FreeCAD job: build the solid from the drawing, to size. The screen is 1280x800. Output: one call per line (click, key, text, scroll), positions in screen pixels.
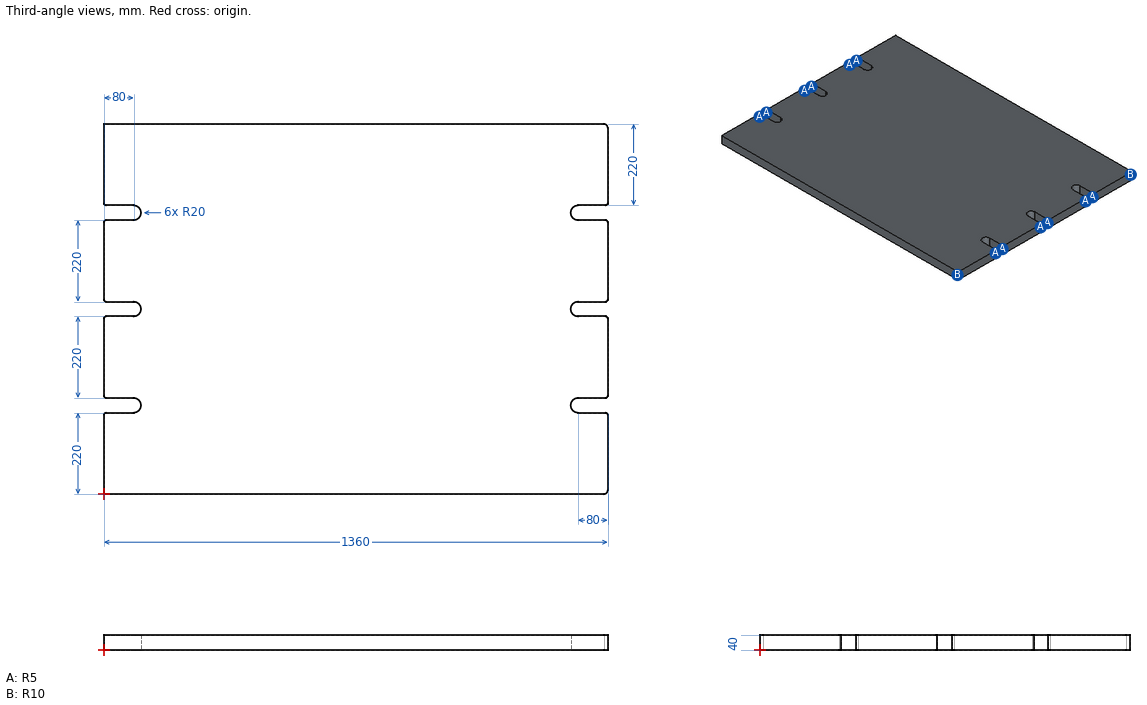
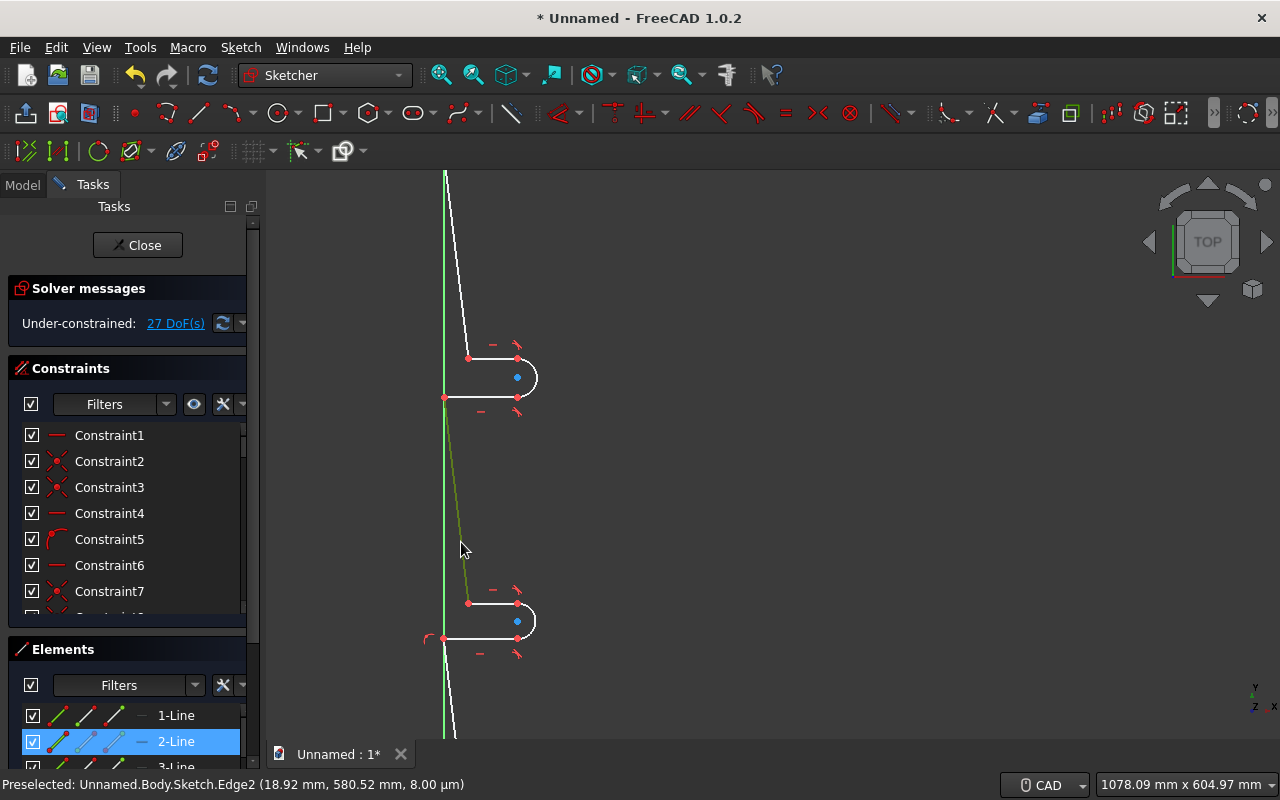
click(668, 114)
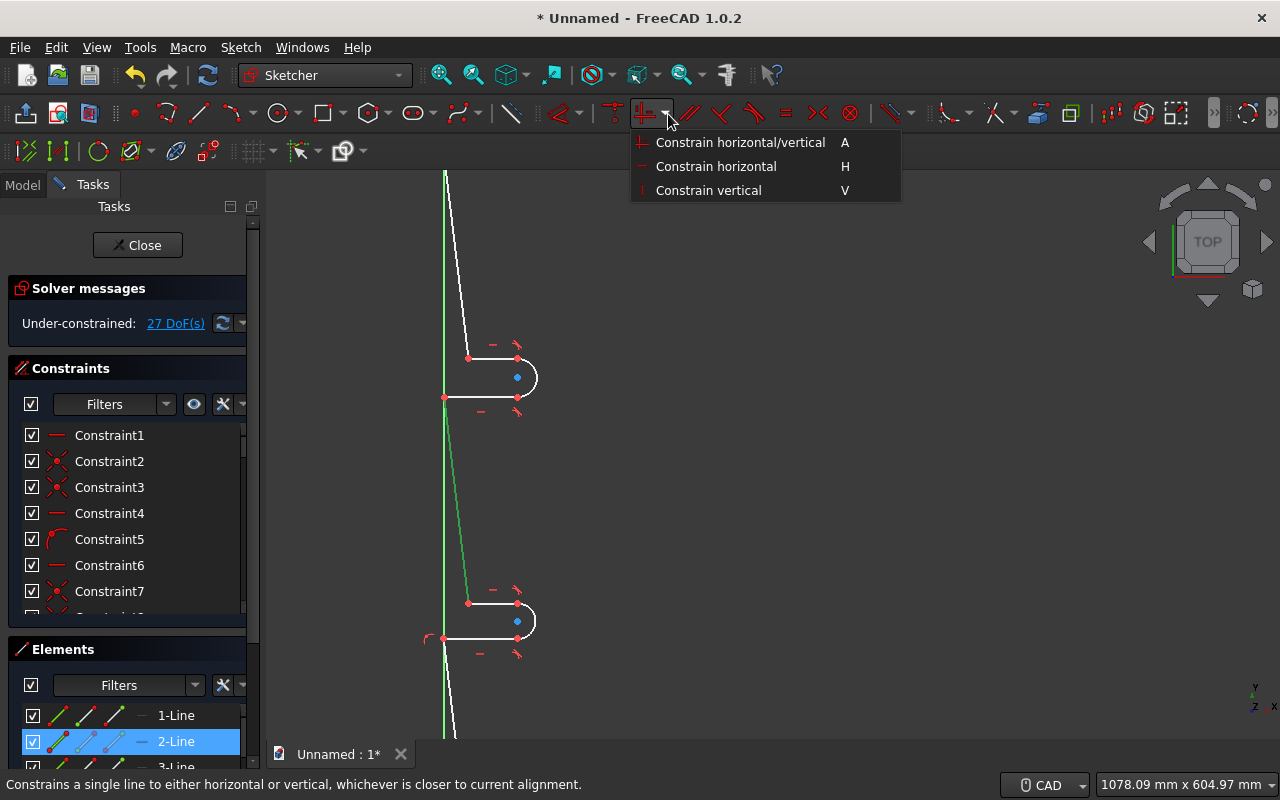
click(766, 190)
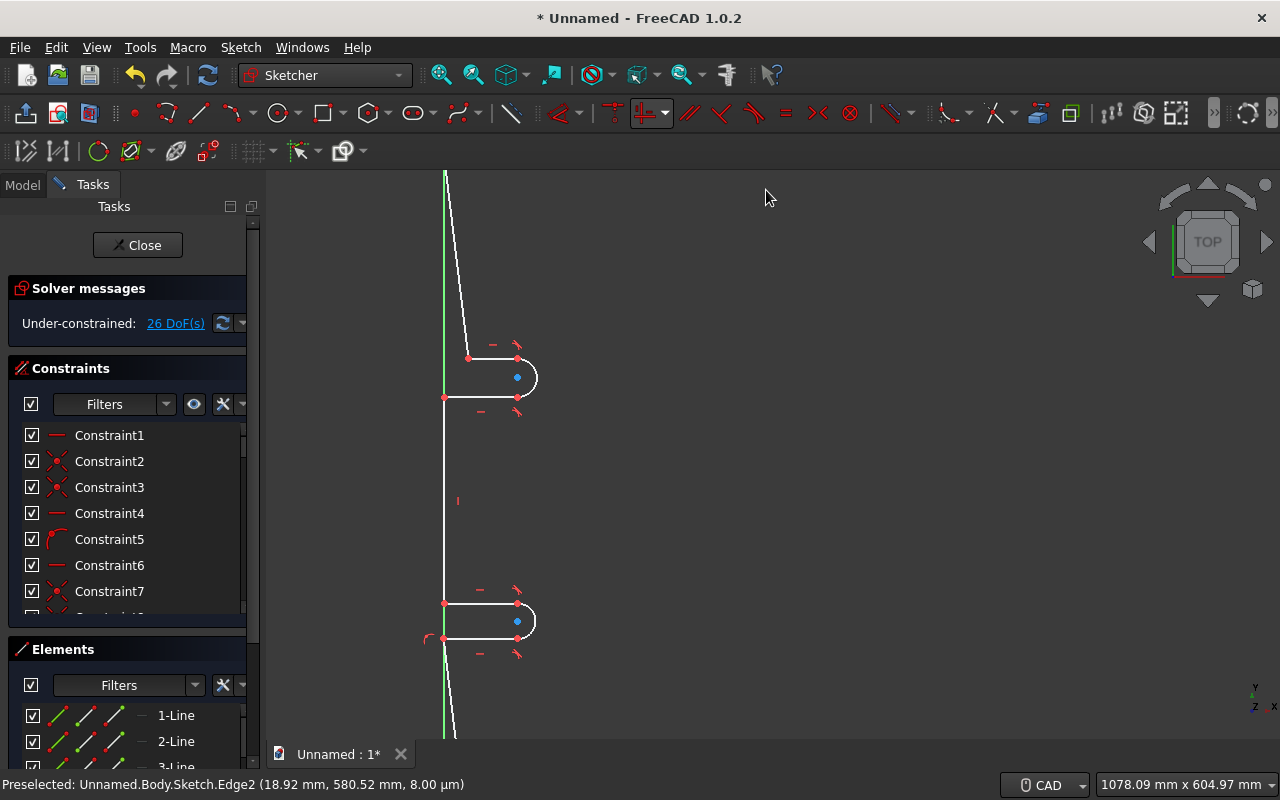
scroll(484, 359, down, 5)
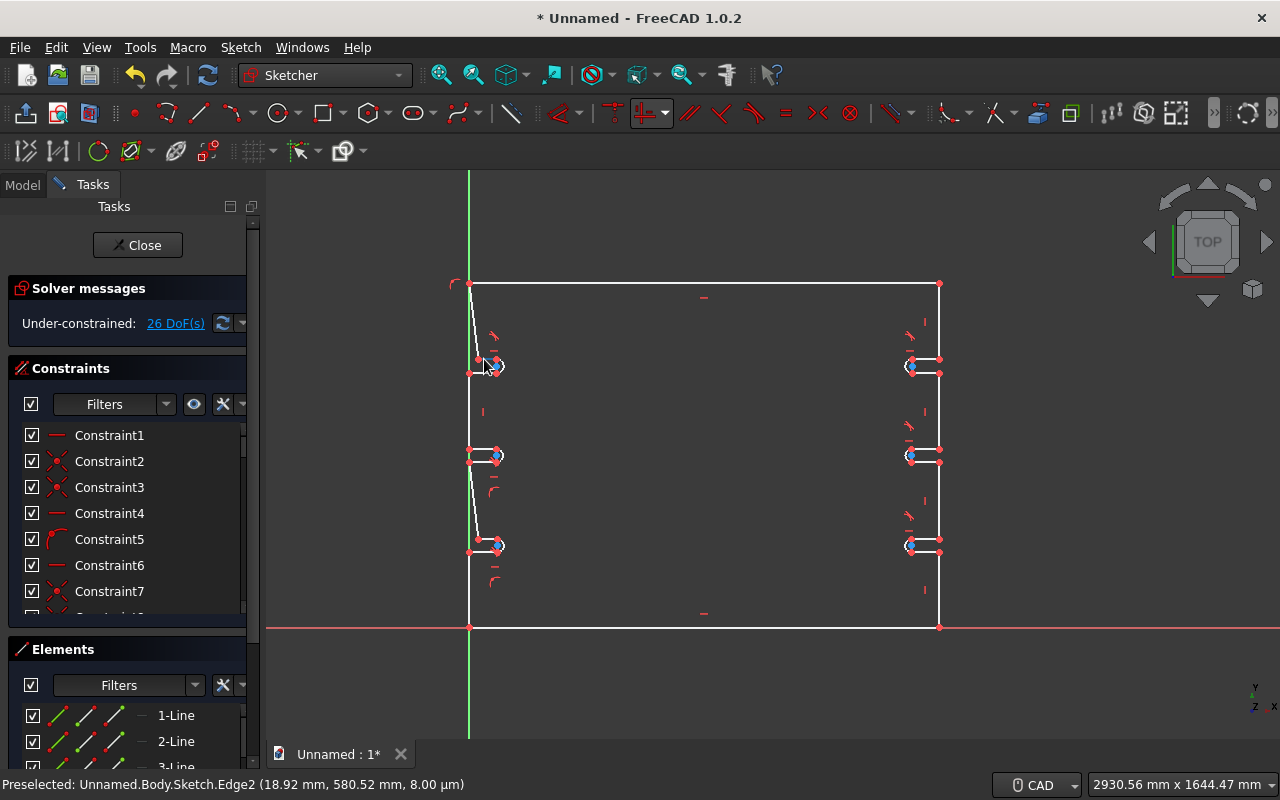
scroll(476, 516, up, 4)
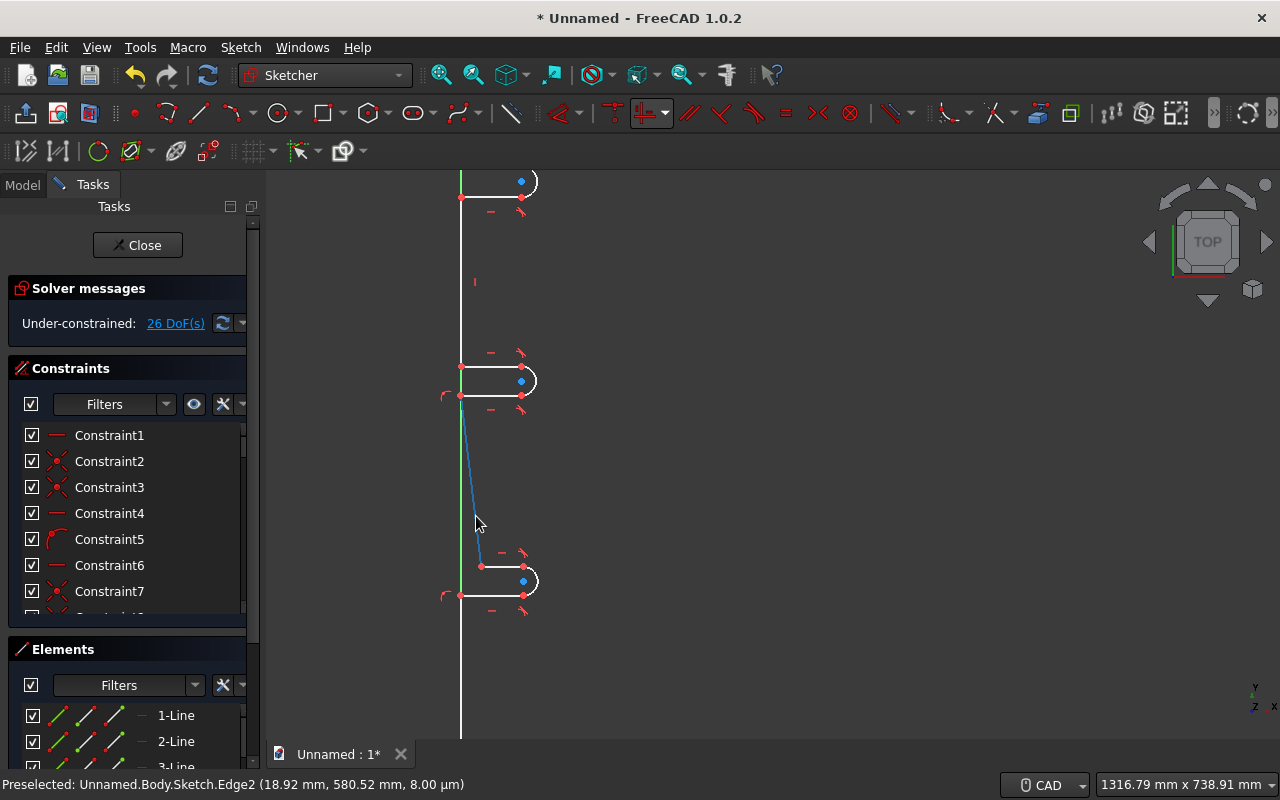
click(475, 515)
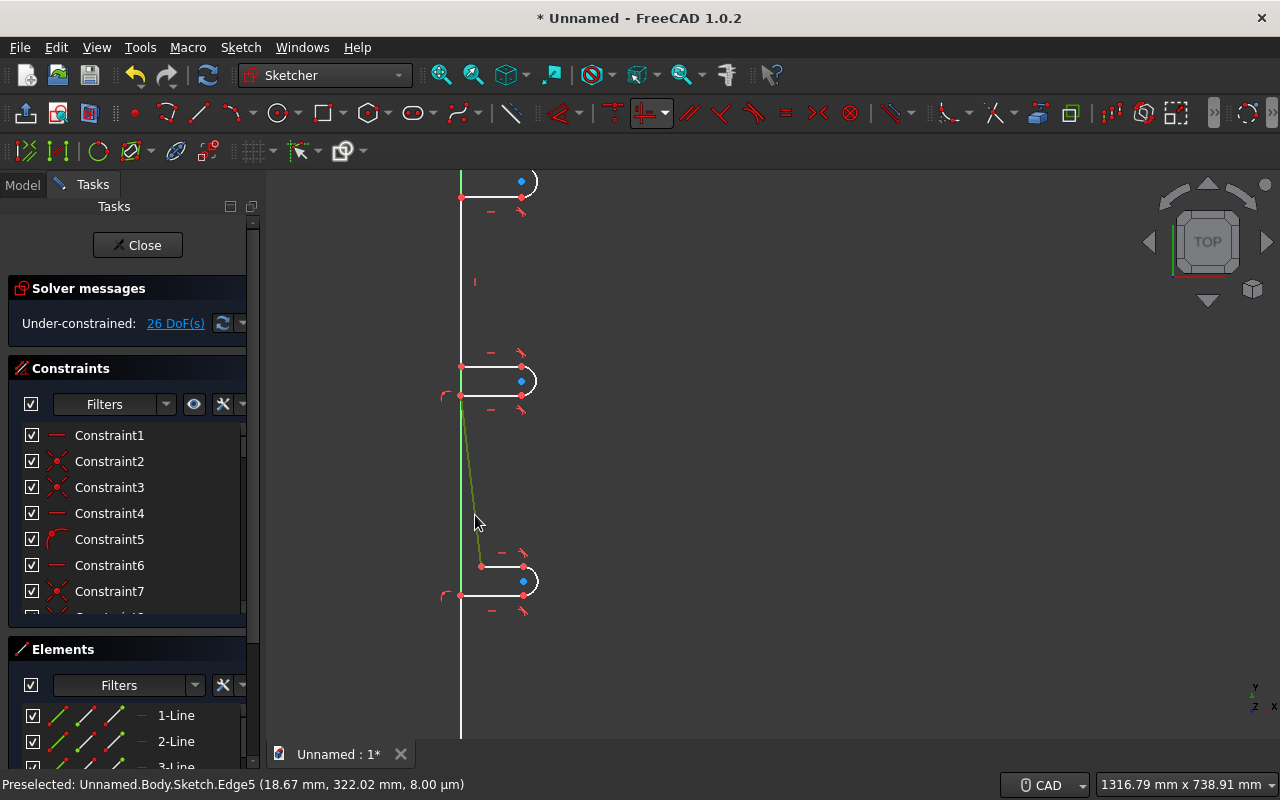
click(668, 114)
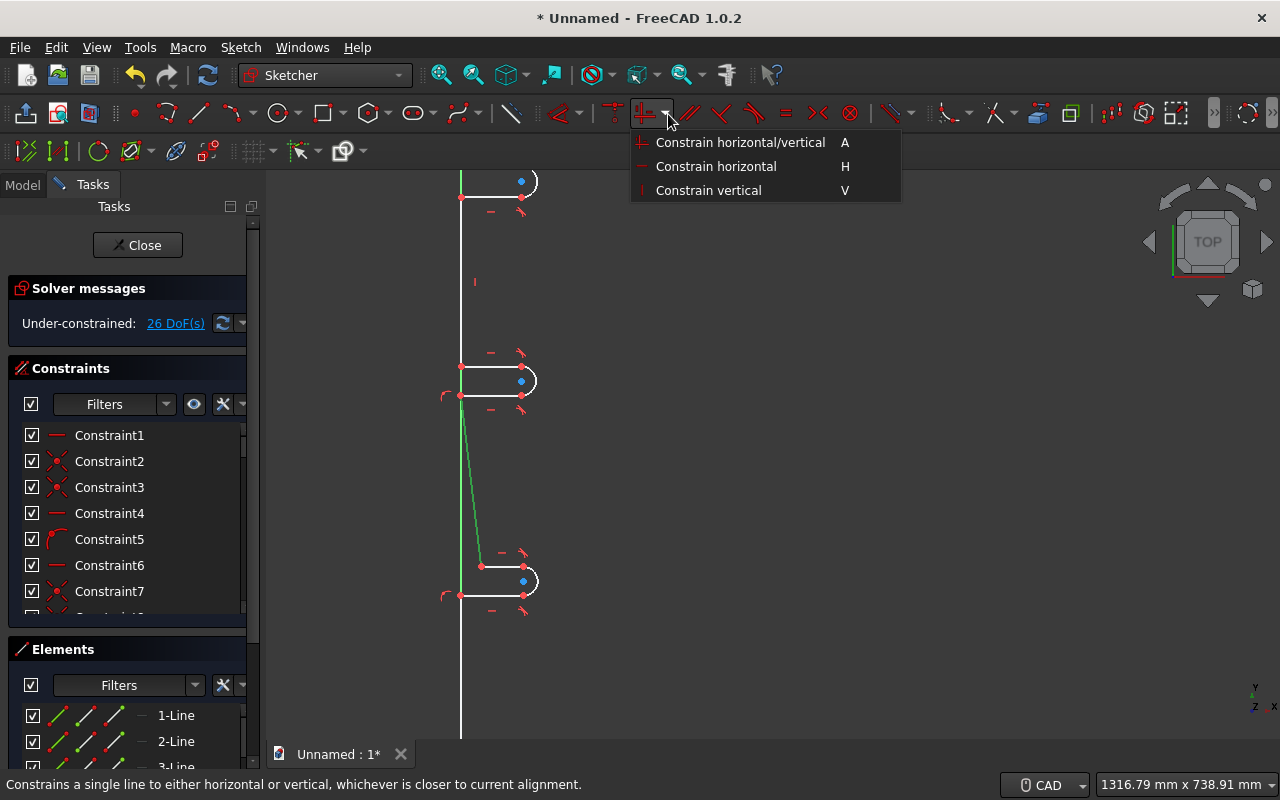
click(766, 190)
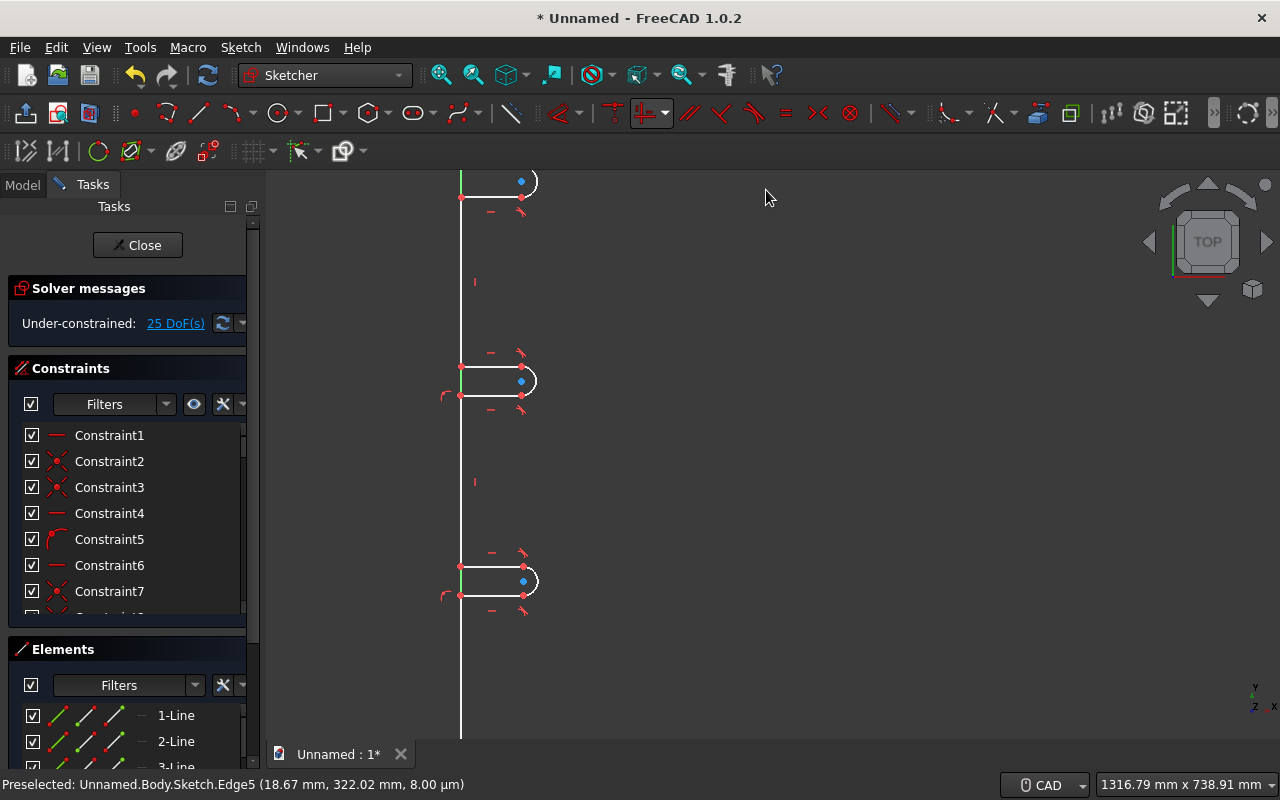
scroll(476, 516, down, 4)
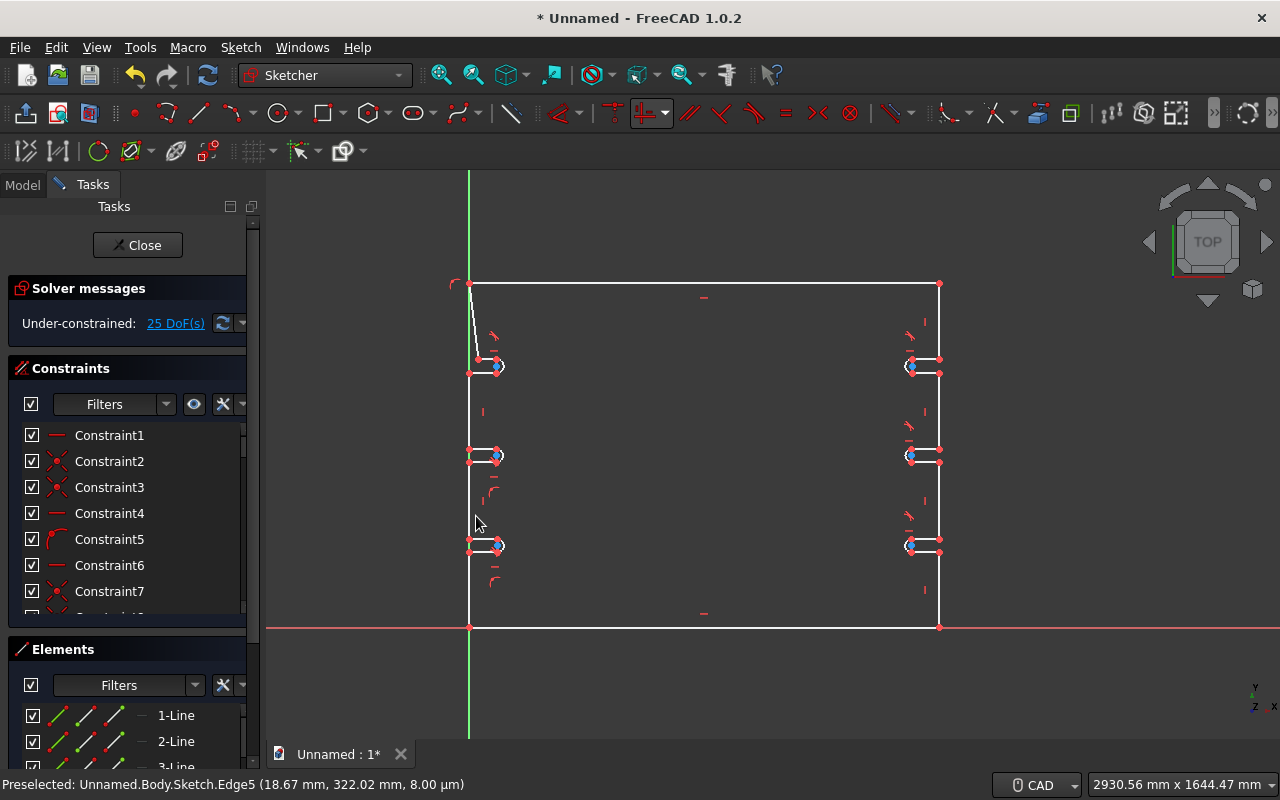
scroll(476, 336, up, 4)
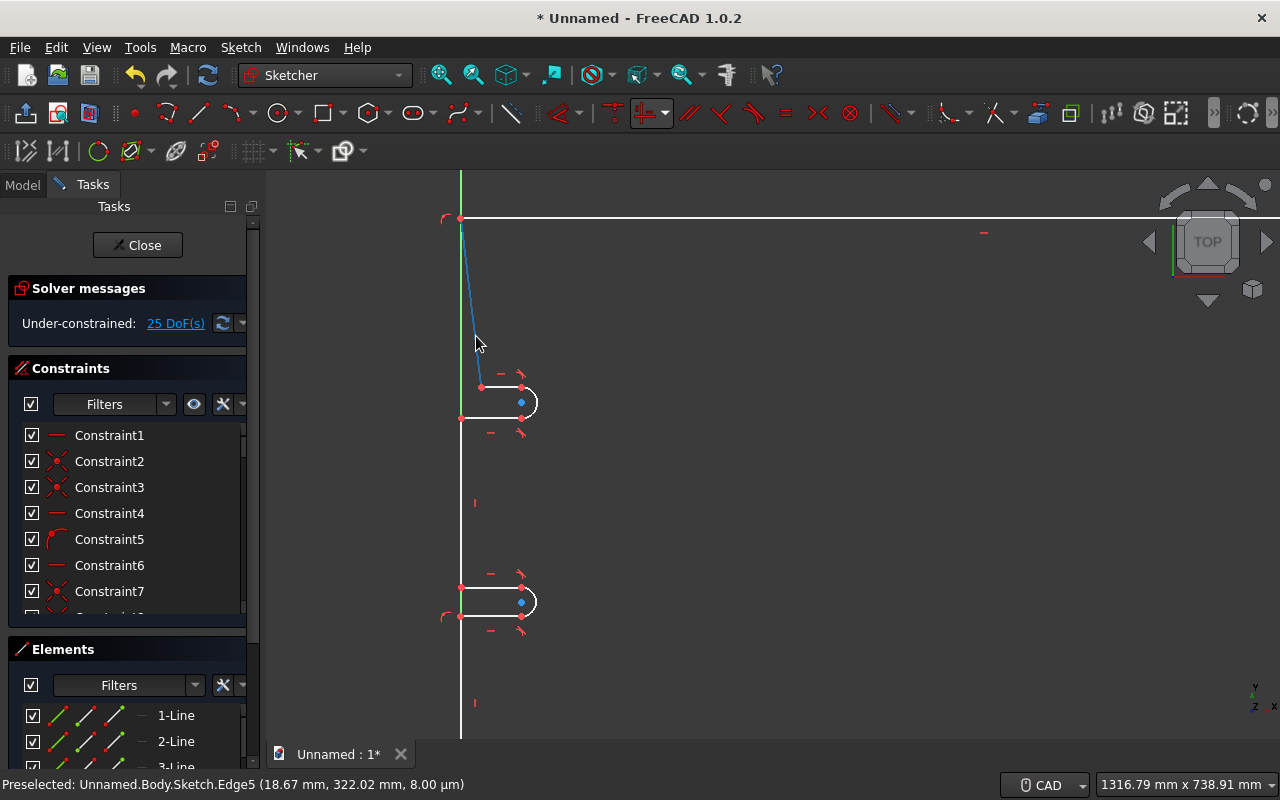
click(475, 337)